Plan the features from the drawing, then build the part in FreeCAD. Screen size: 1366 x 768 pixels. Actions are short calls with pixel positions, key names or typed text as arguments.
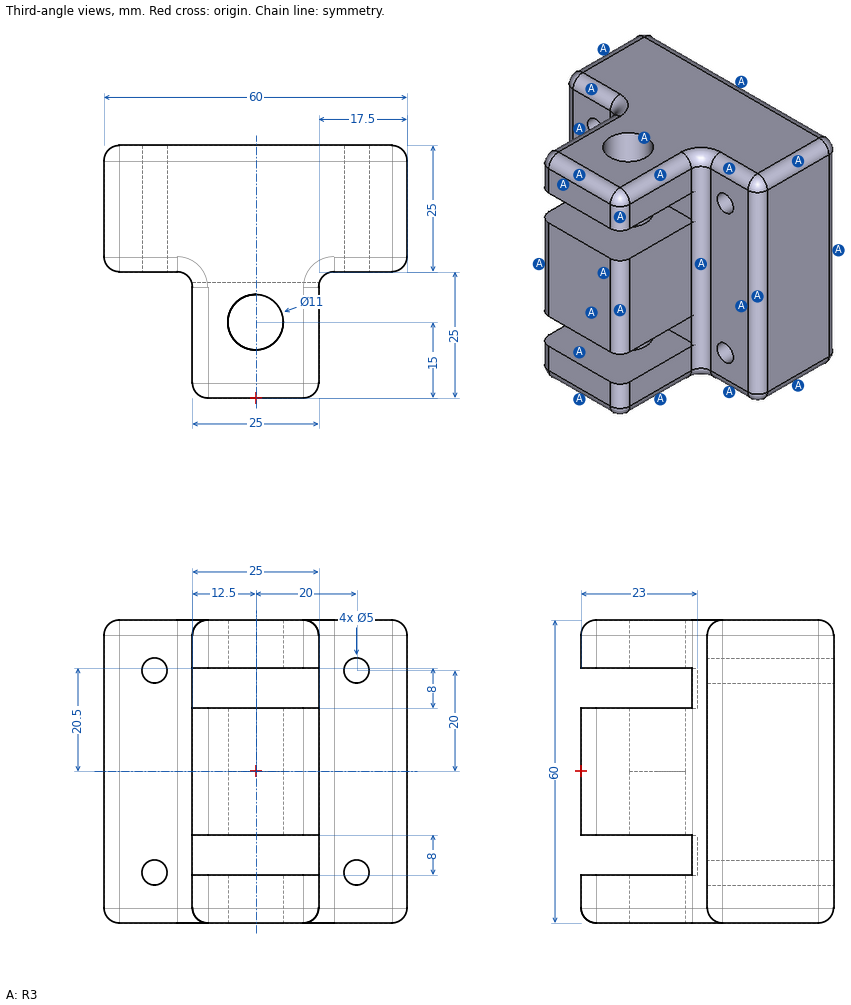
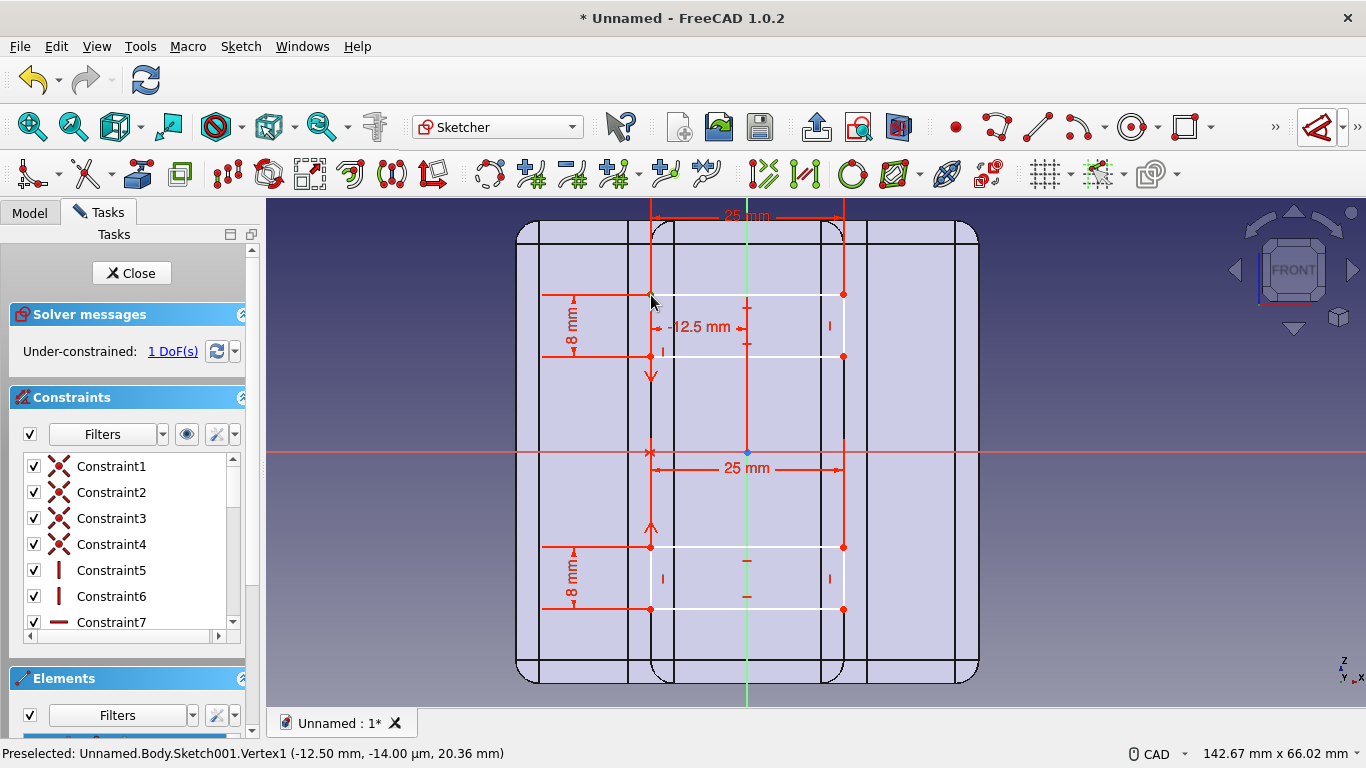
click(1342, 128)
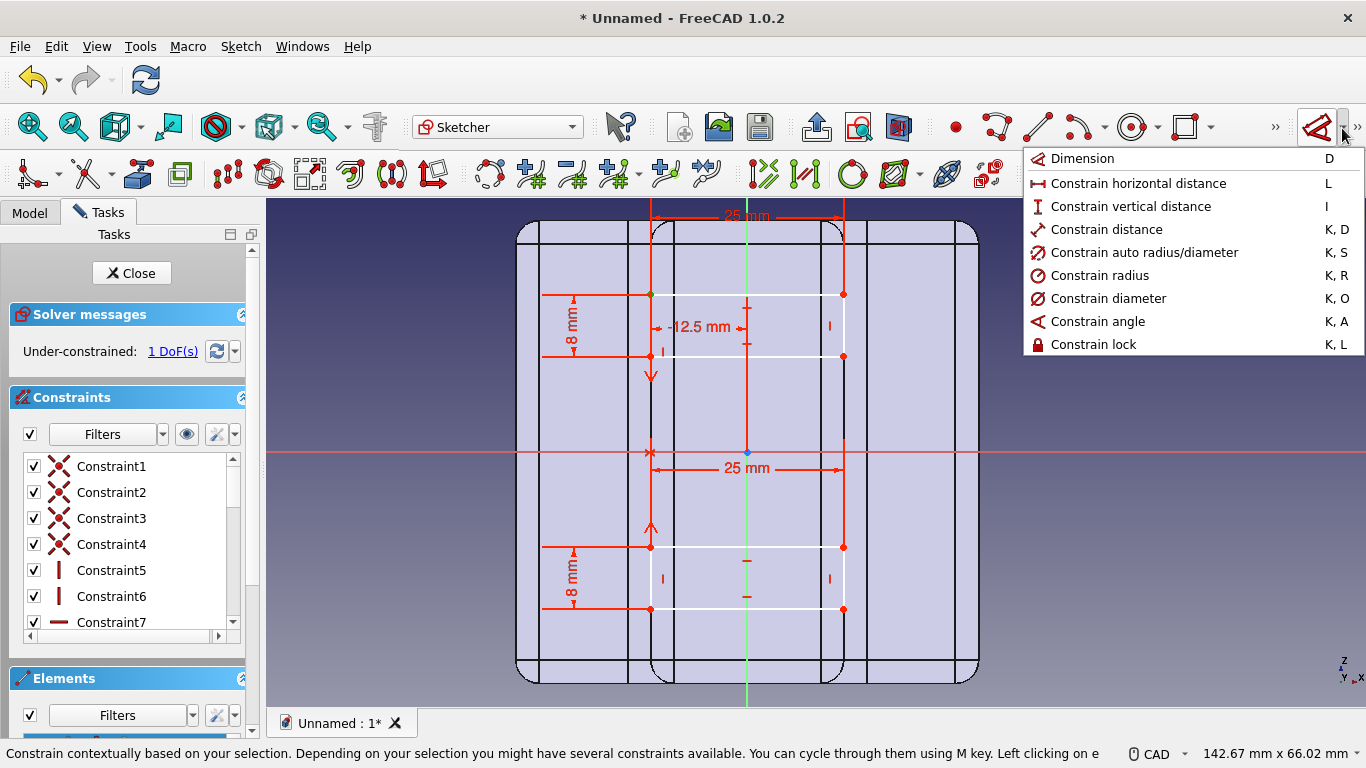
click(1194, 206)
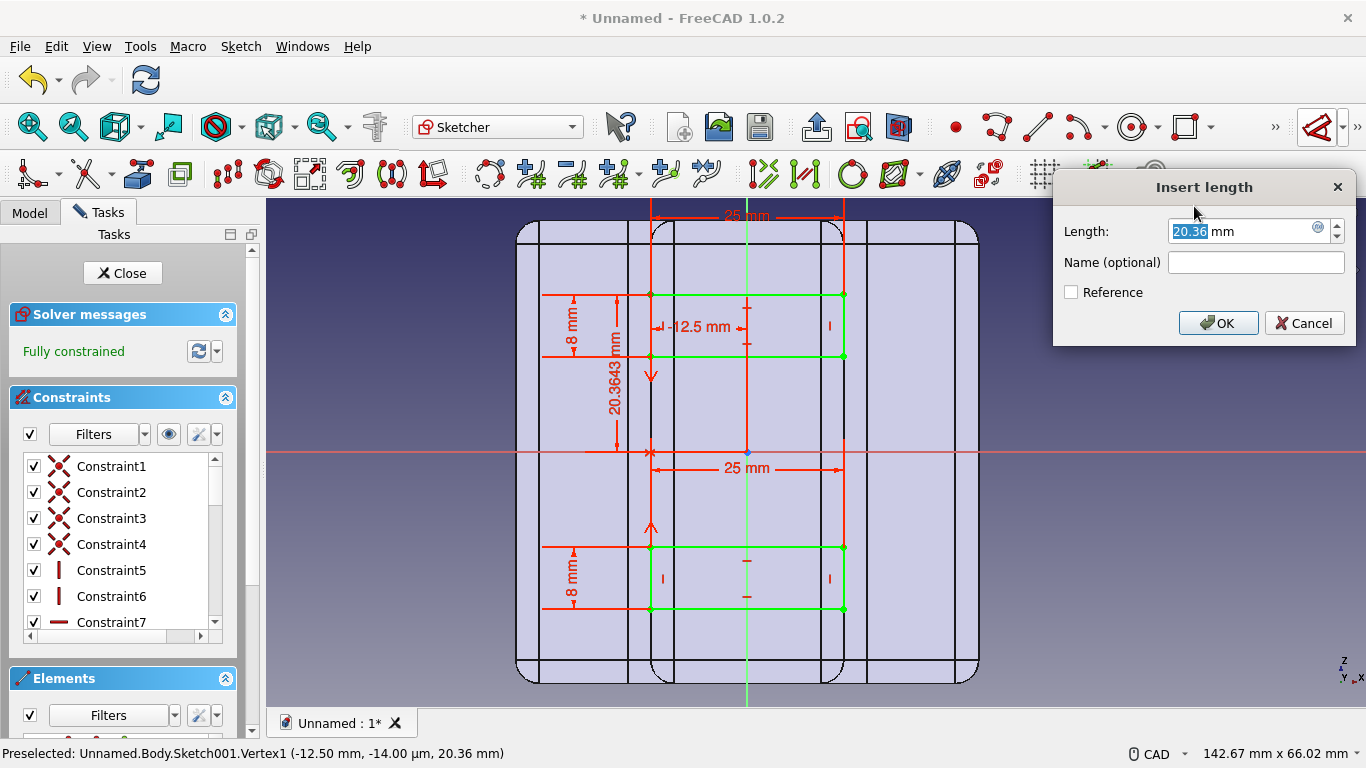
text(20.5)
key(Return)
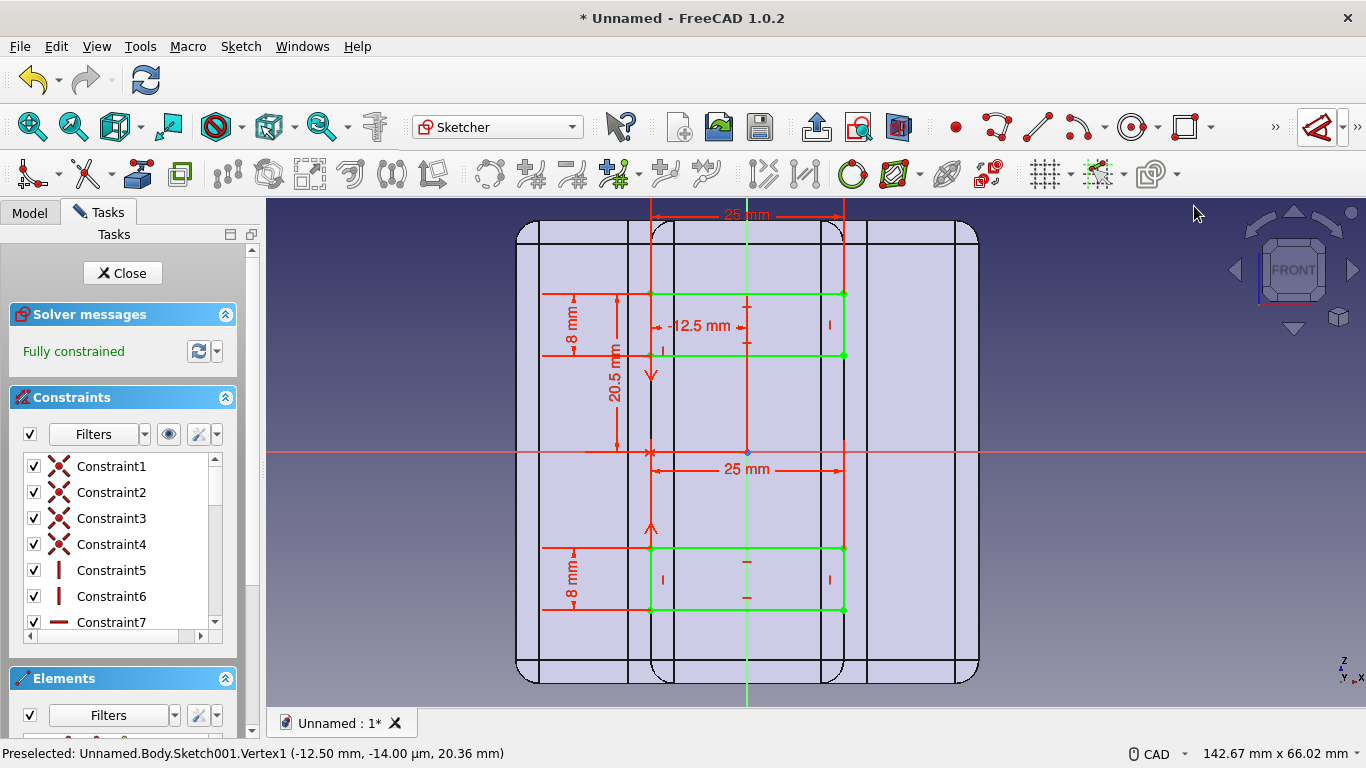
click(123, 273)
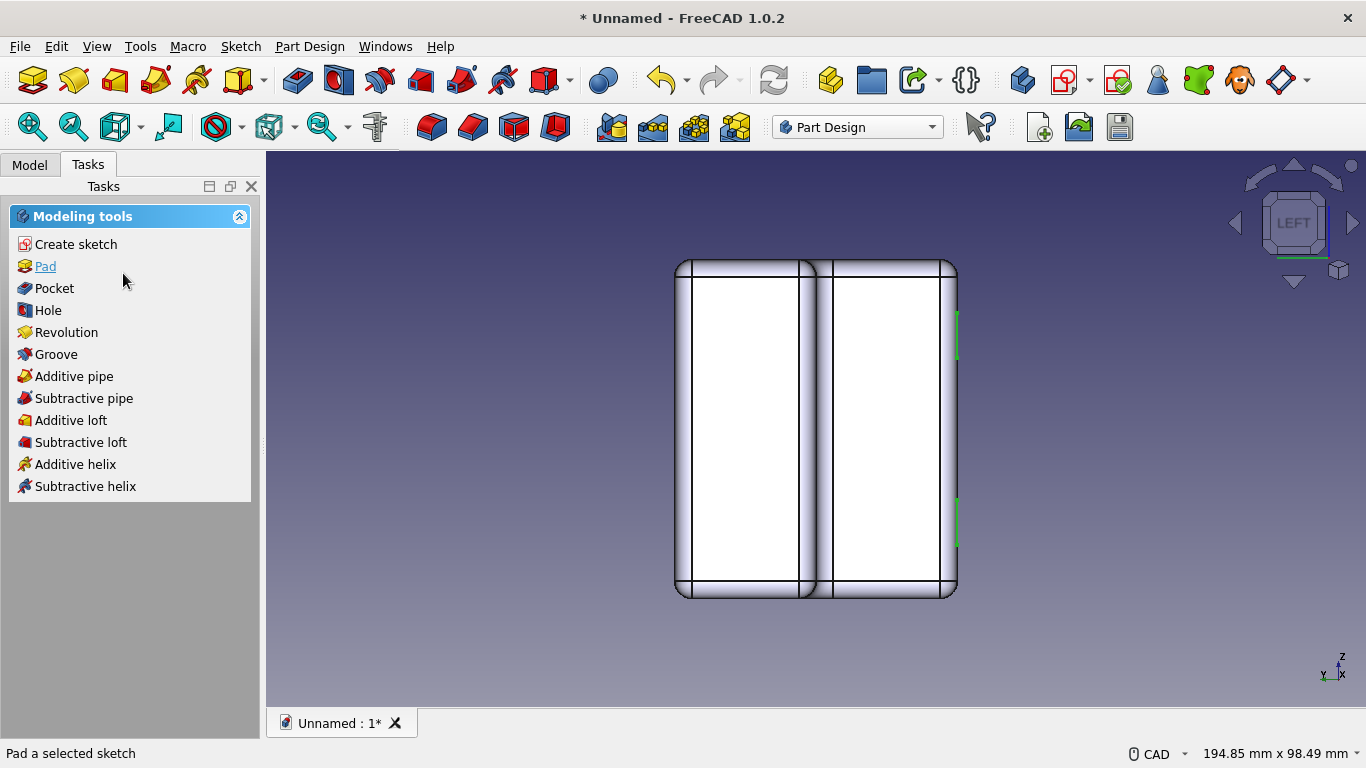
click(298, 80)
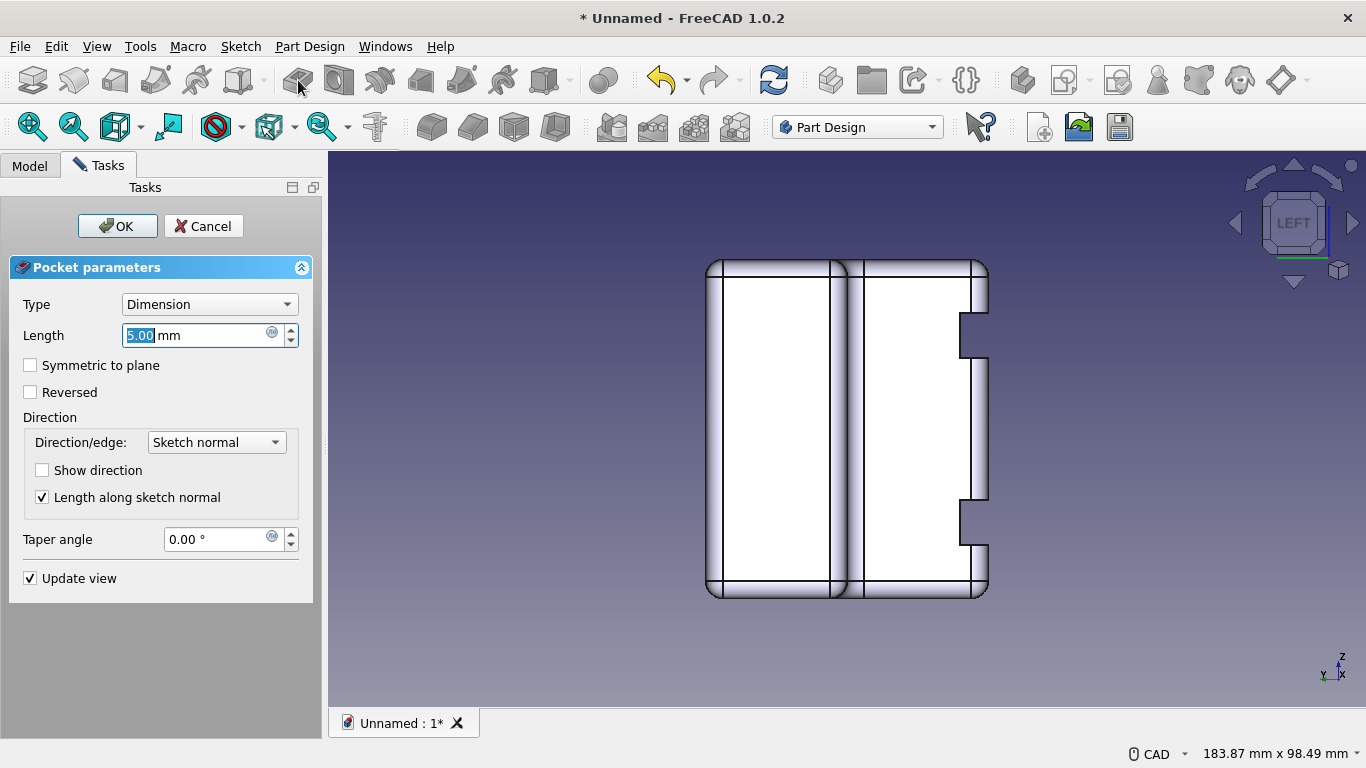
text(23)
key(Tab)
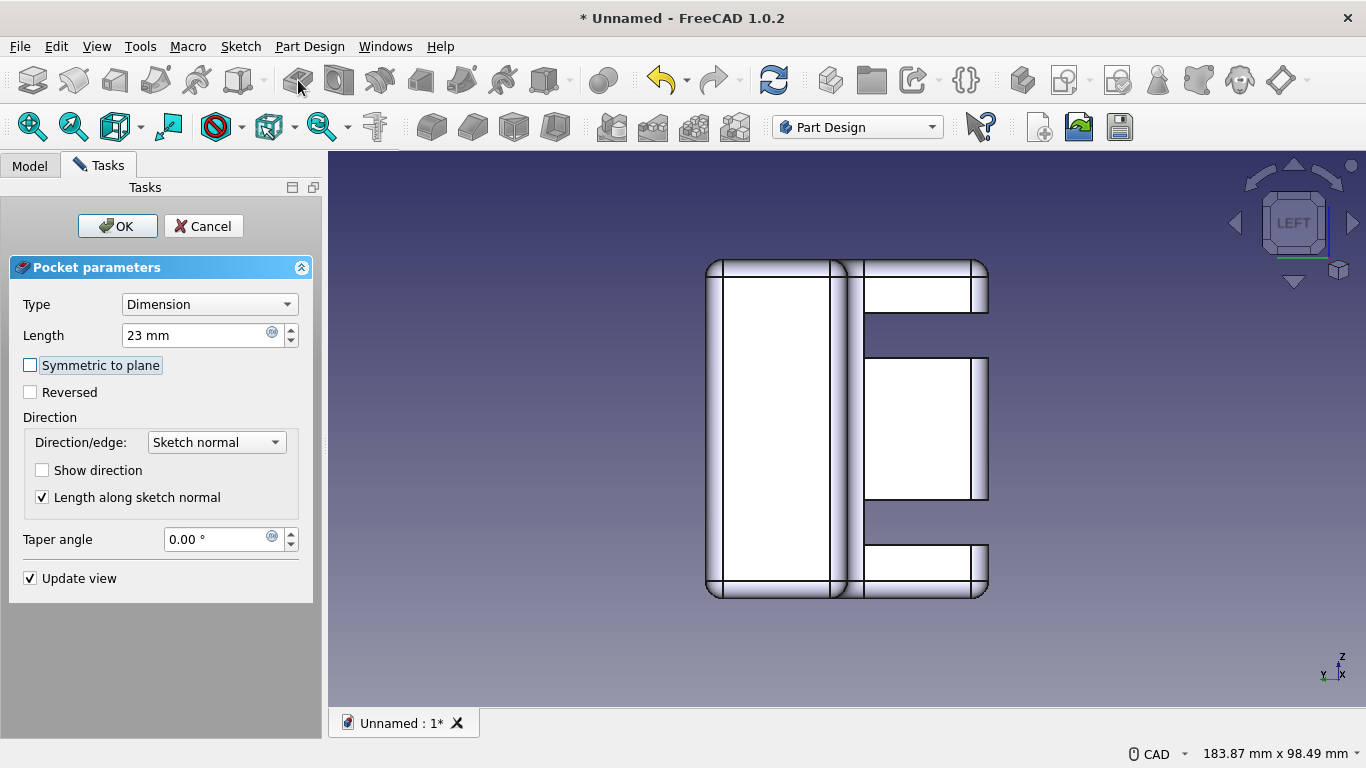
click(118, 226)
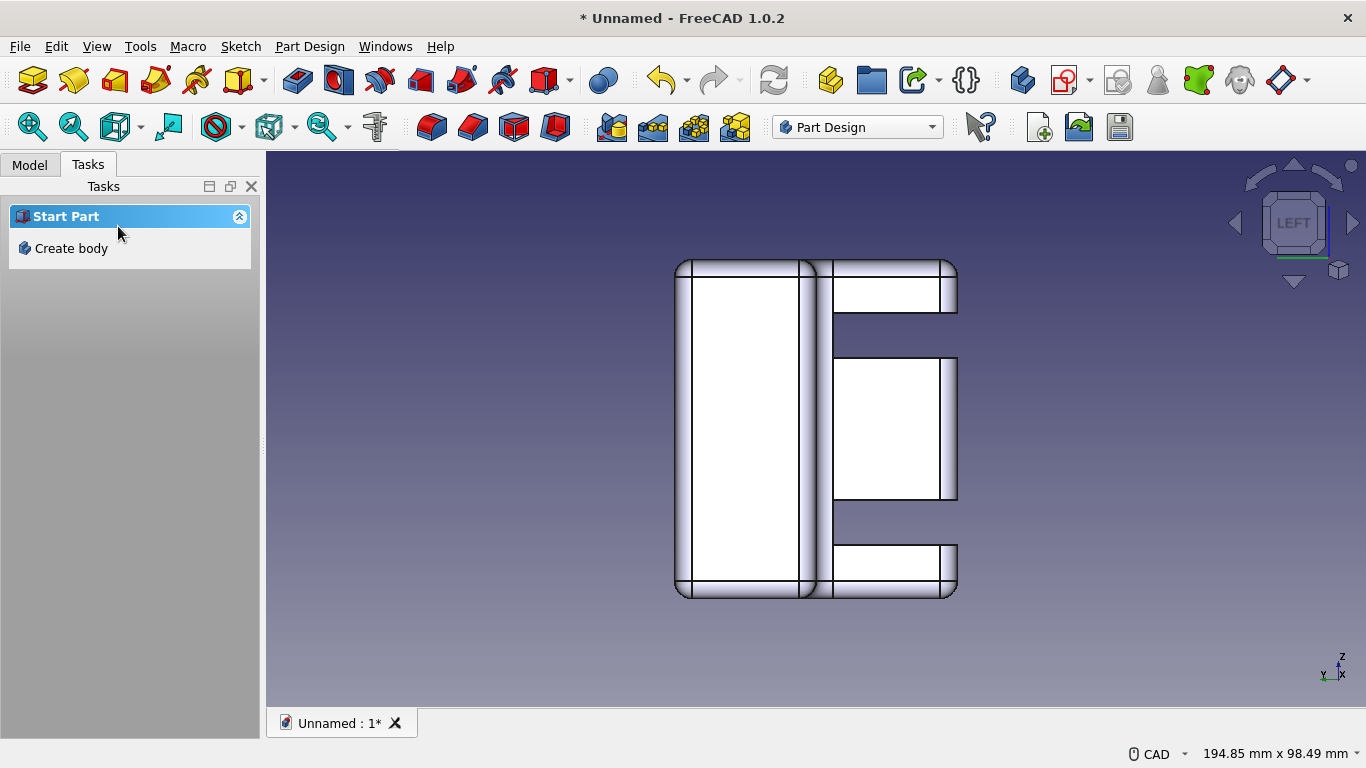
key(0)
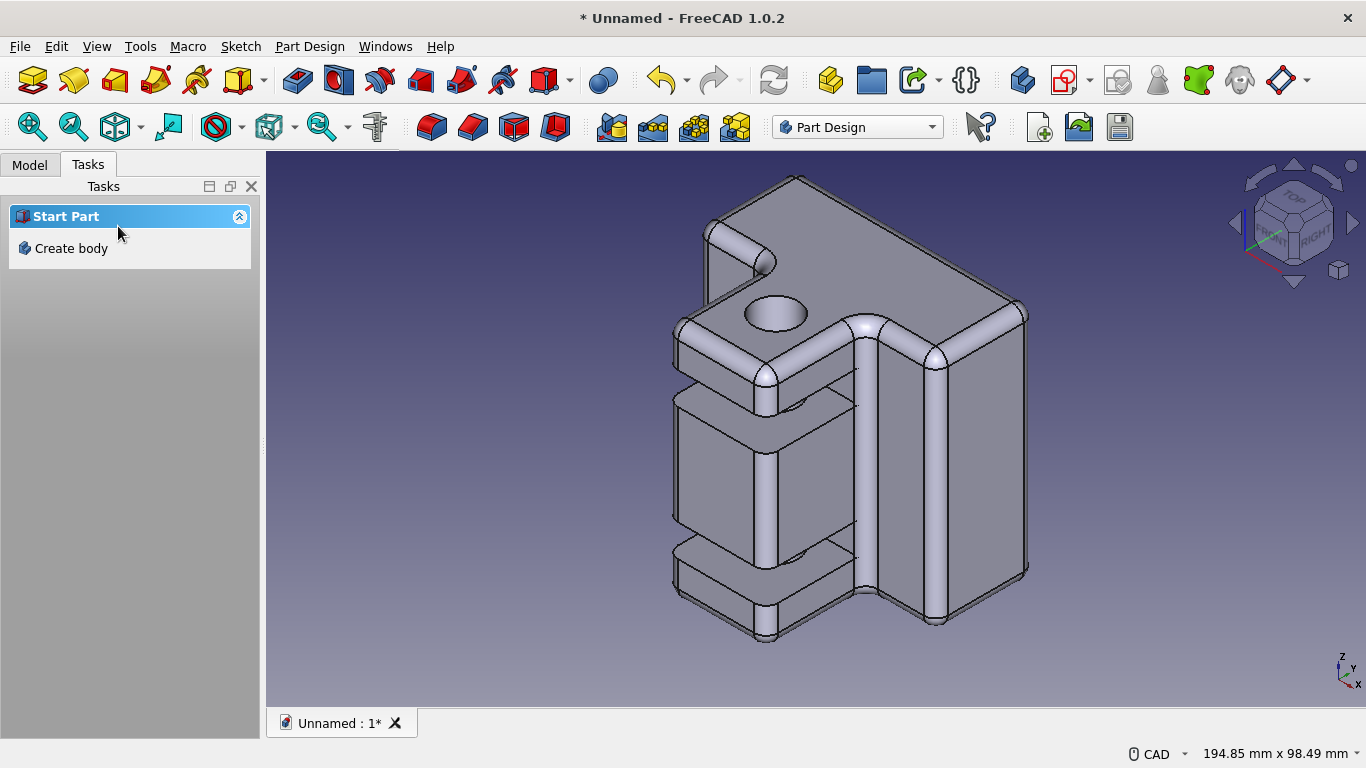
click(901, 406)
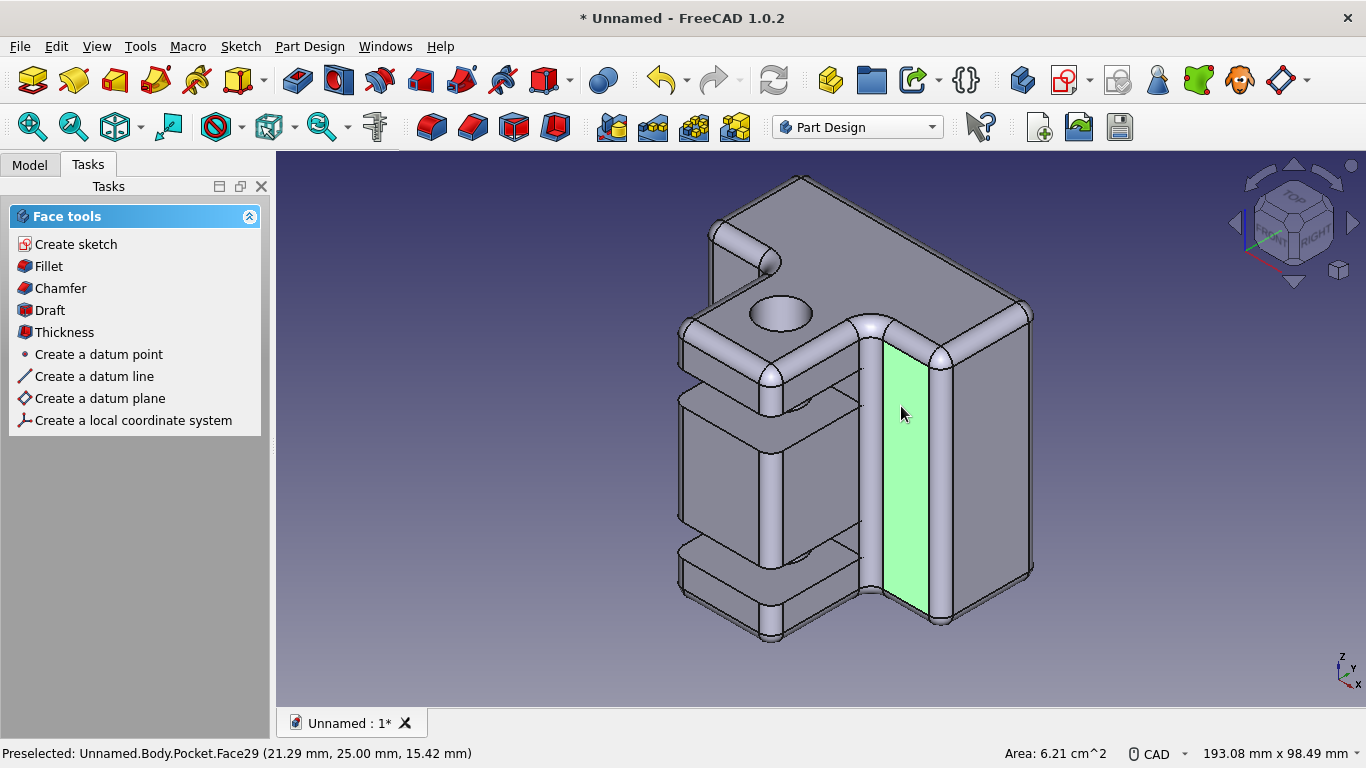
click(1064, 80)